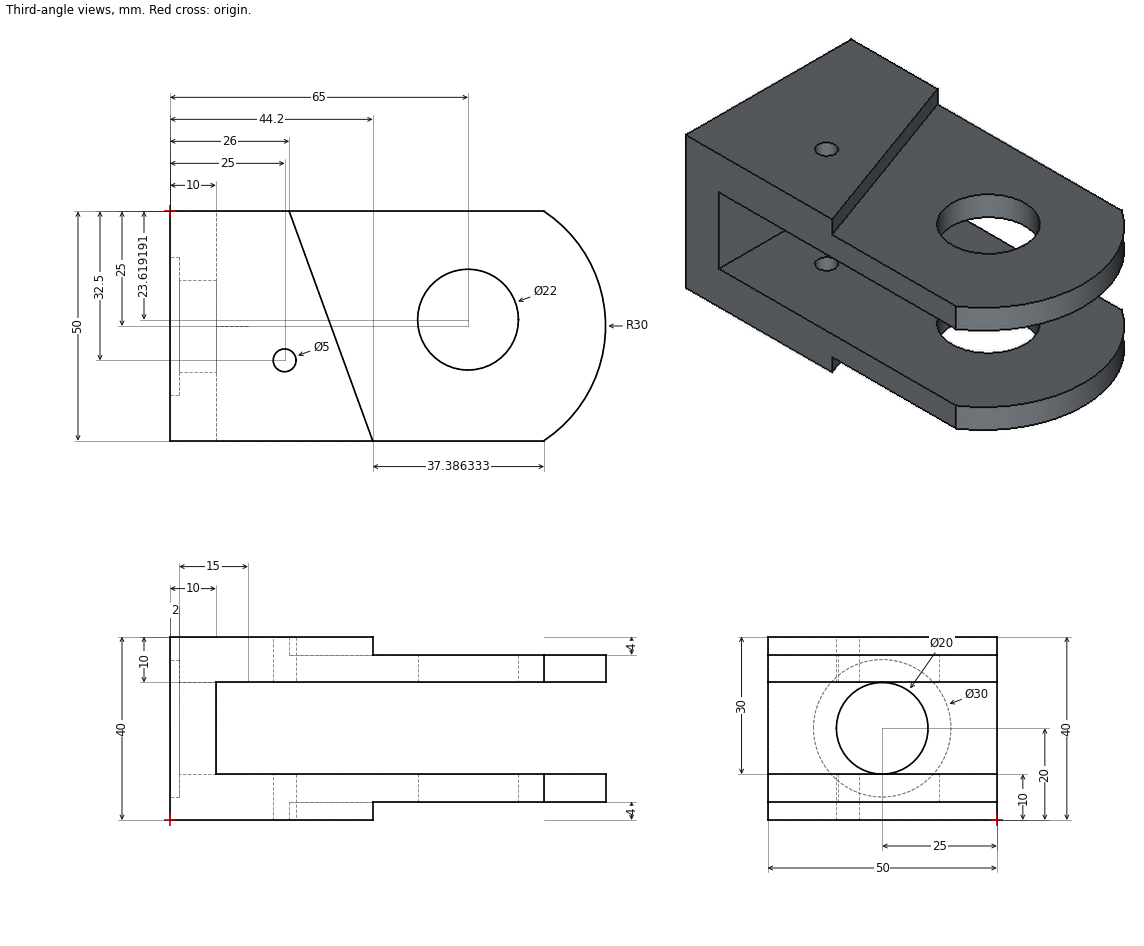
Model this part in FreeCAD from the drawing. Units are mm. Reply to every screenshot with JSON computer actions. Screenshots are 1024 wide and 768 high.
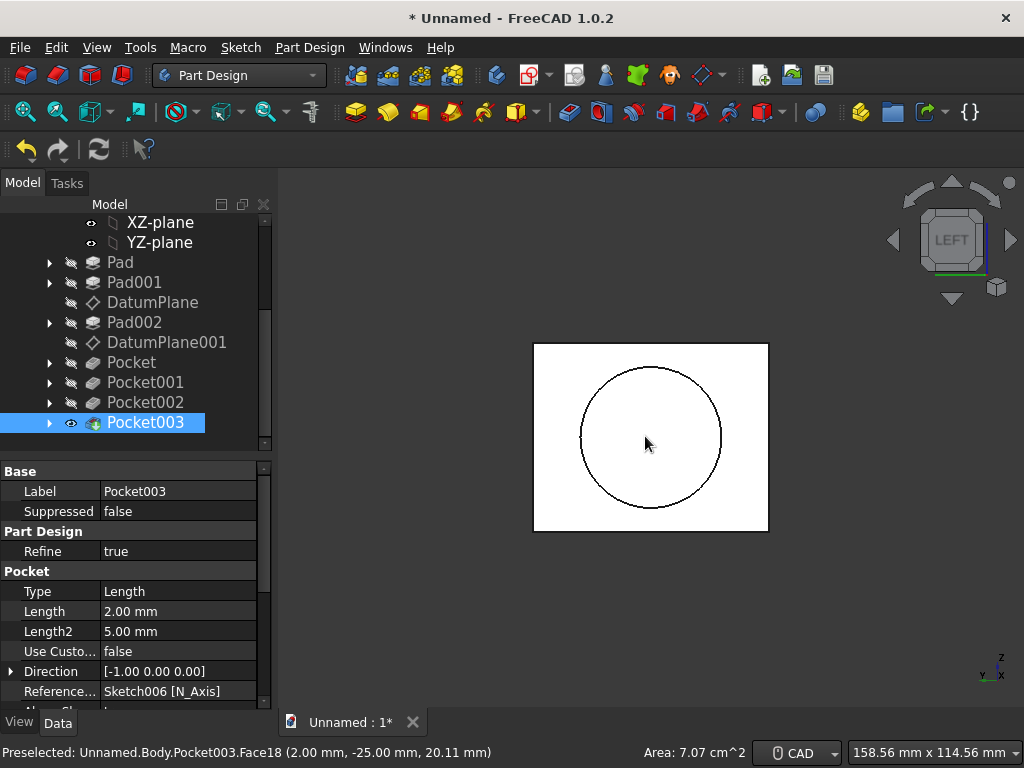
{"action": "left_click", "coordinate": [530, 76]}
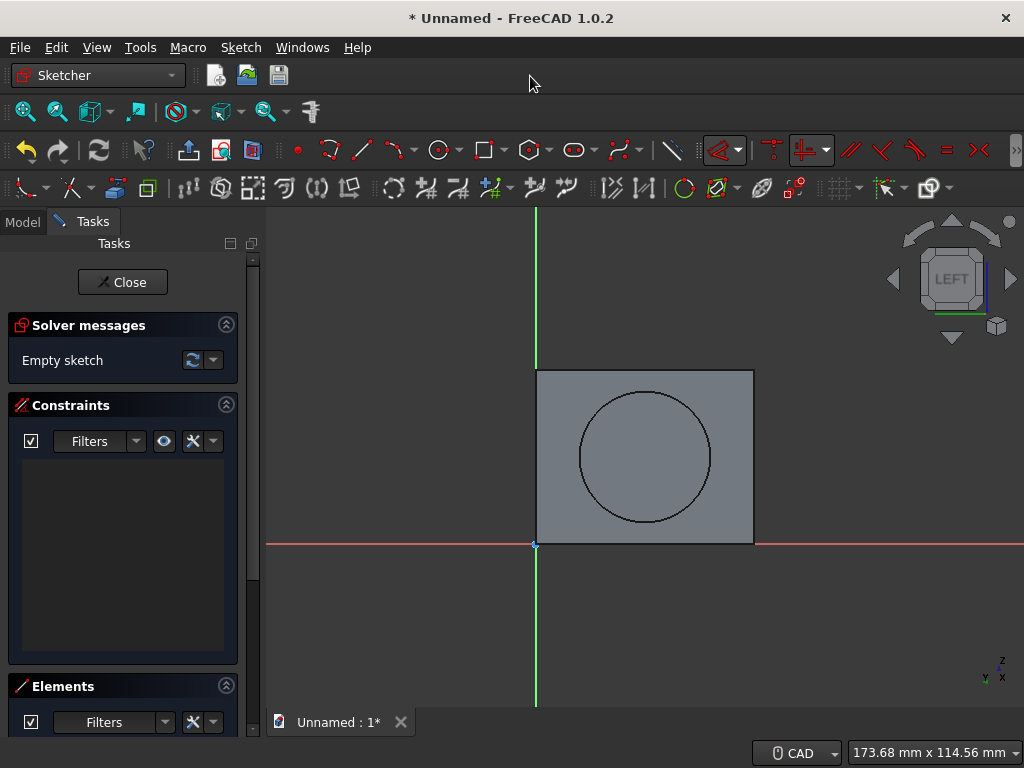
{"action": "left_click", "coordinate": [254, 150]}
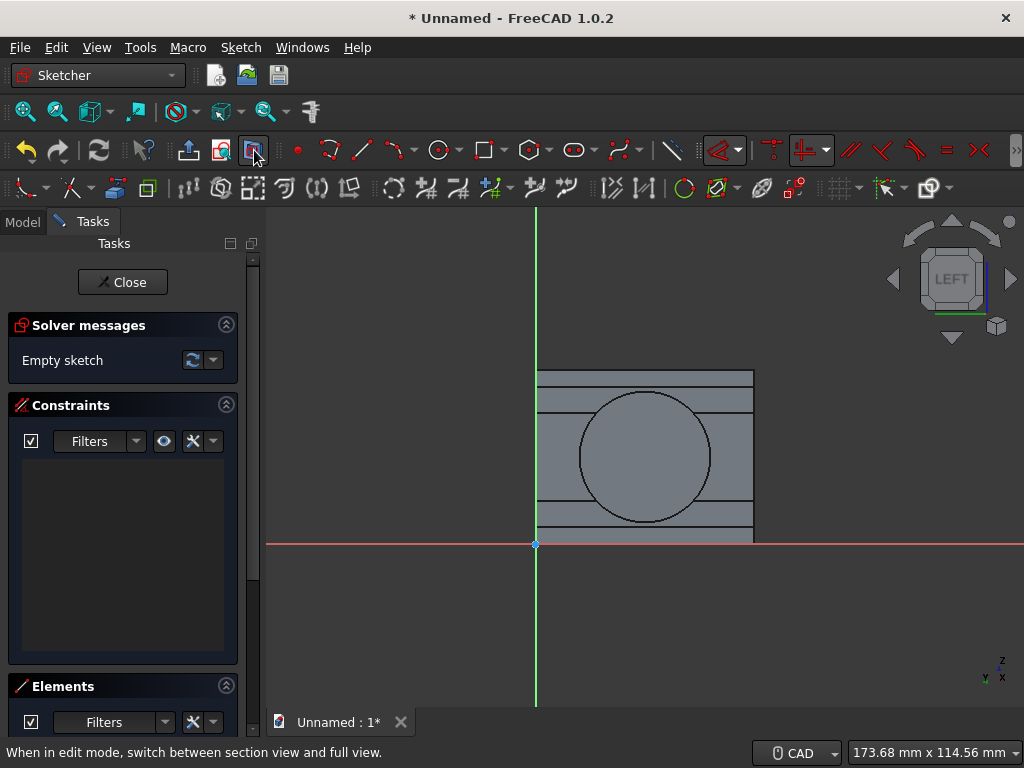
{"action": "scroll", "coordinate": [641, 497], "scroll_direction": "up", "scroll_amount": 4}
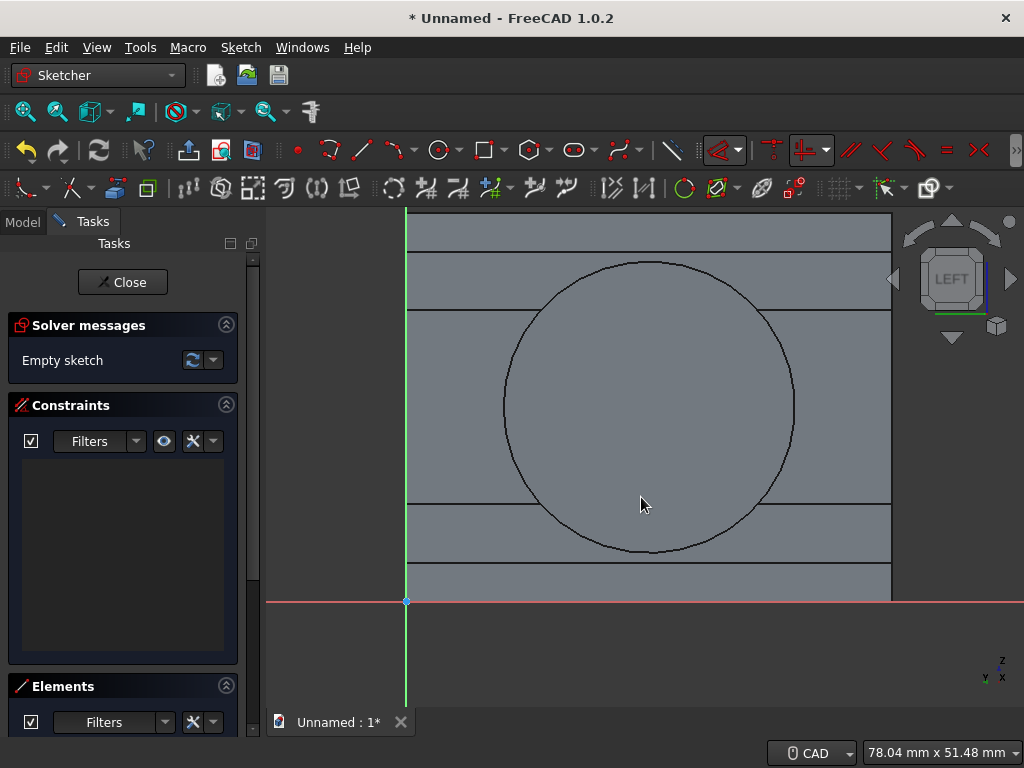
{"action": "left_click", "coordinate": [440, 150]}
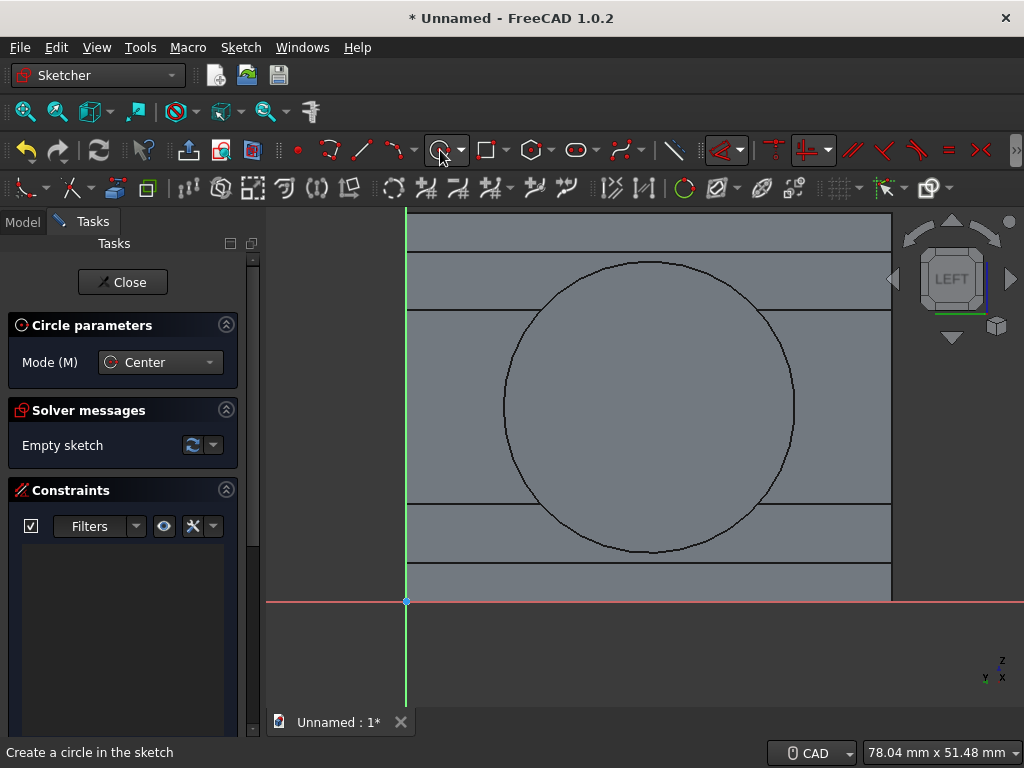
{"action": "left_click", "coordinate": [649, 407]}
{"action": "mouse_move", "coordinate": [718, 339]}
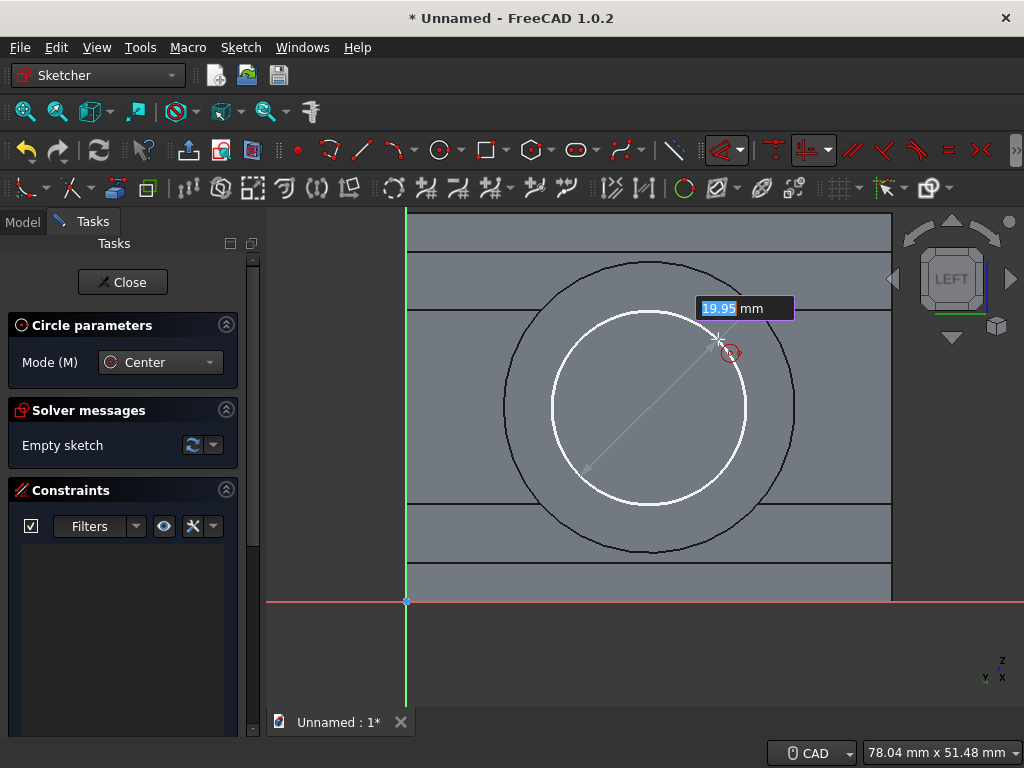
{"action": "type", "text": "20"}
{"action": "key", "text": "Return"}
{"action": "key", "text": "Escape"}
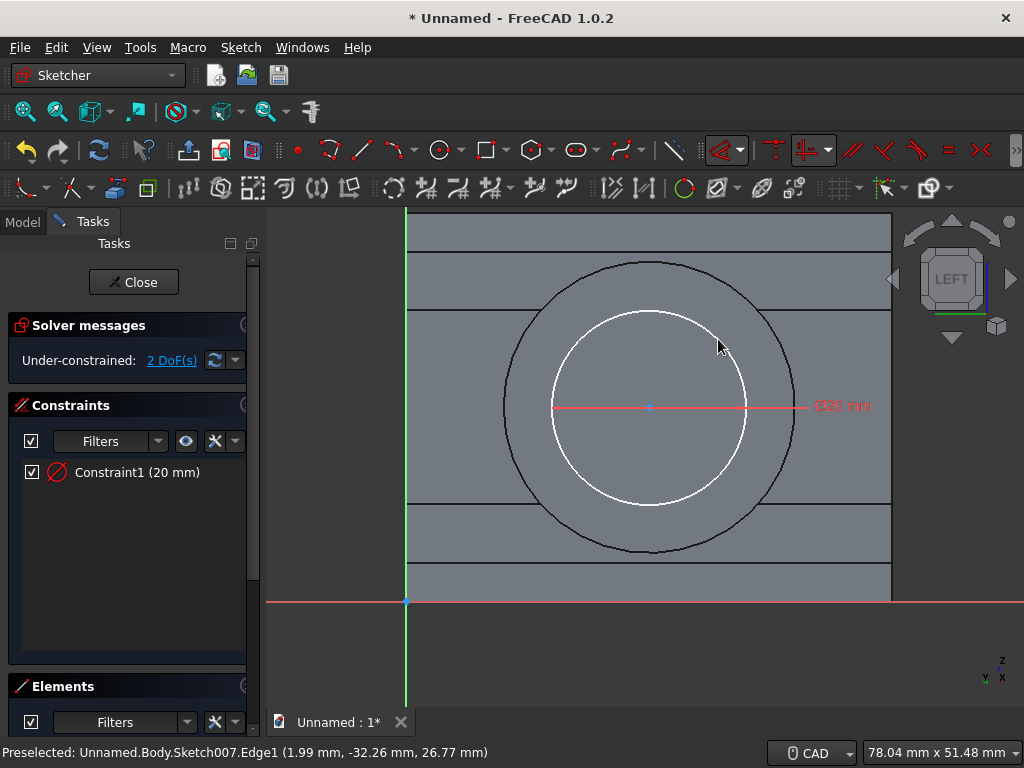
{"action": "left_click", "coordinate": [649, 408]}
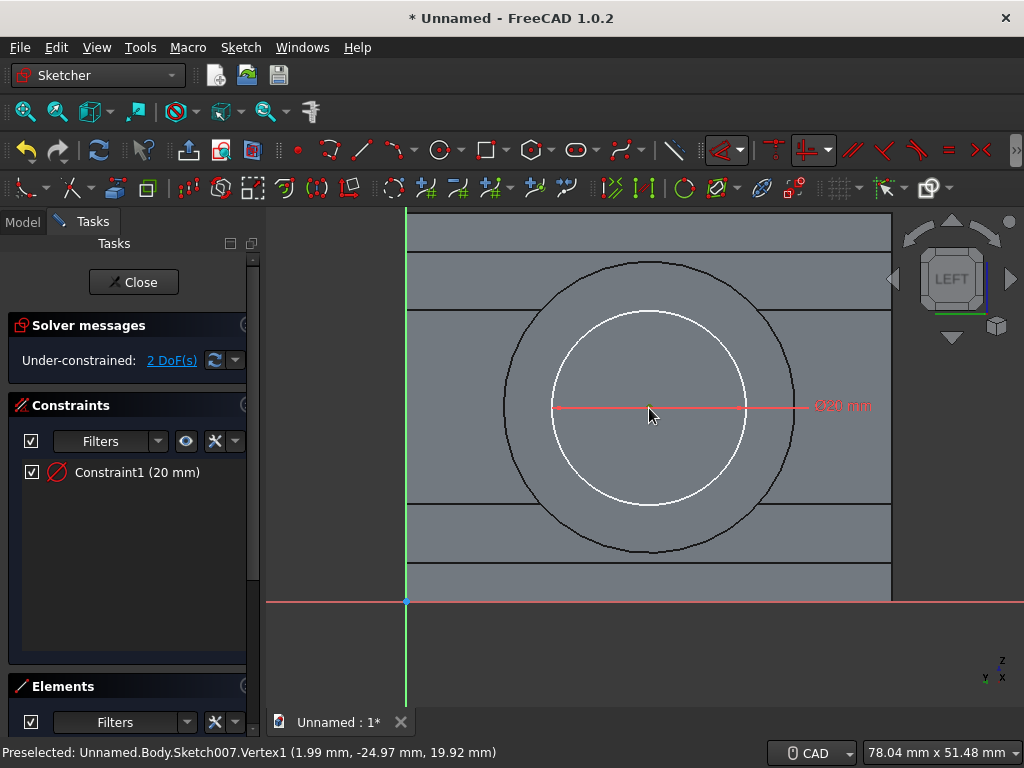
{"action": "left_click", "coordinate": [742, 150]}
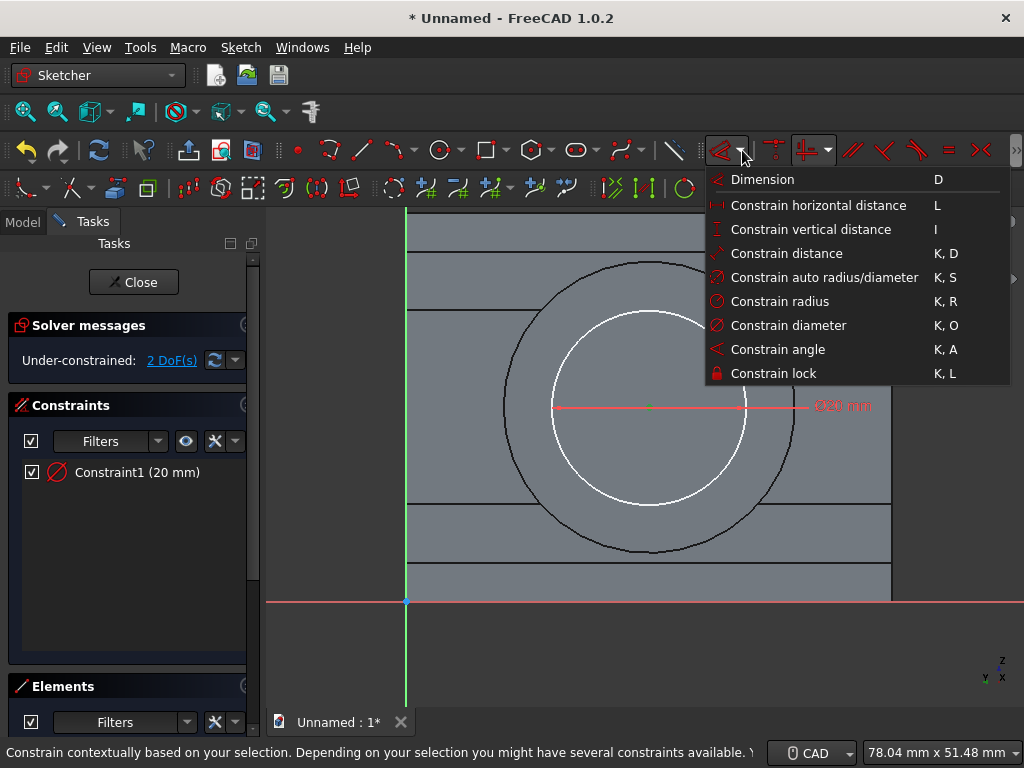
{"action": "left_click", "coordinate": [858, 205]}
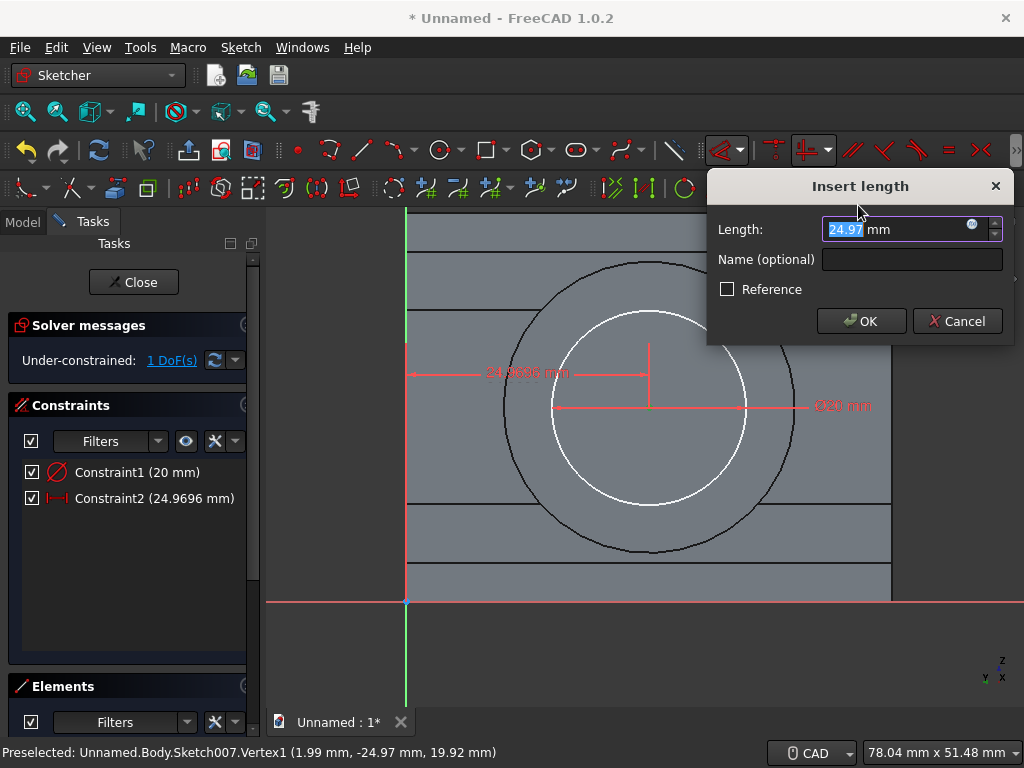
{"action": "type", "text": "25"}
{"action": "key", "text": "Return"}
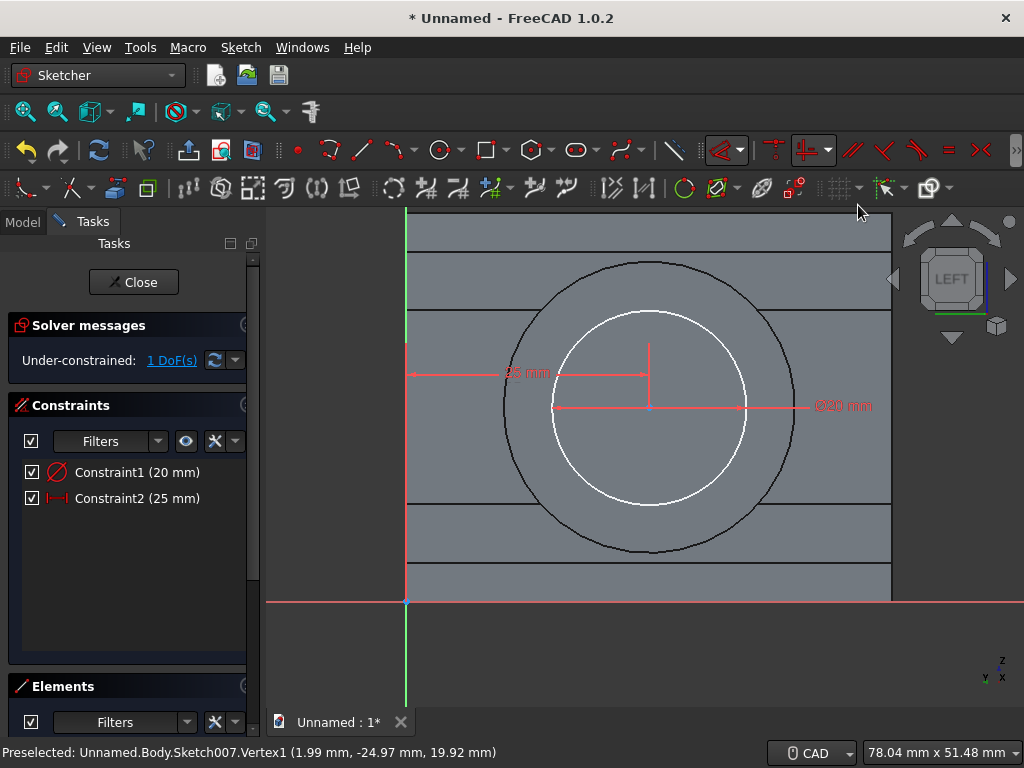
{"action": "left_click", "coordinate": [649, 408]}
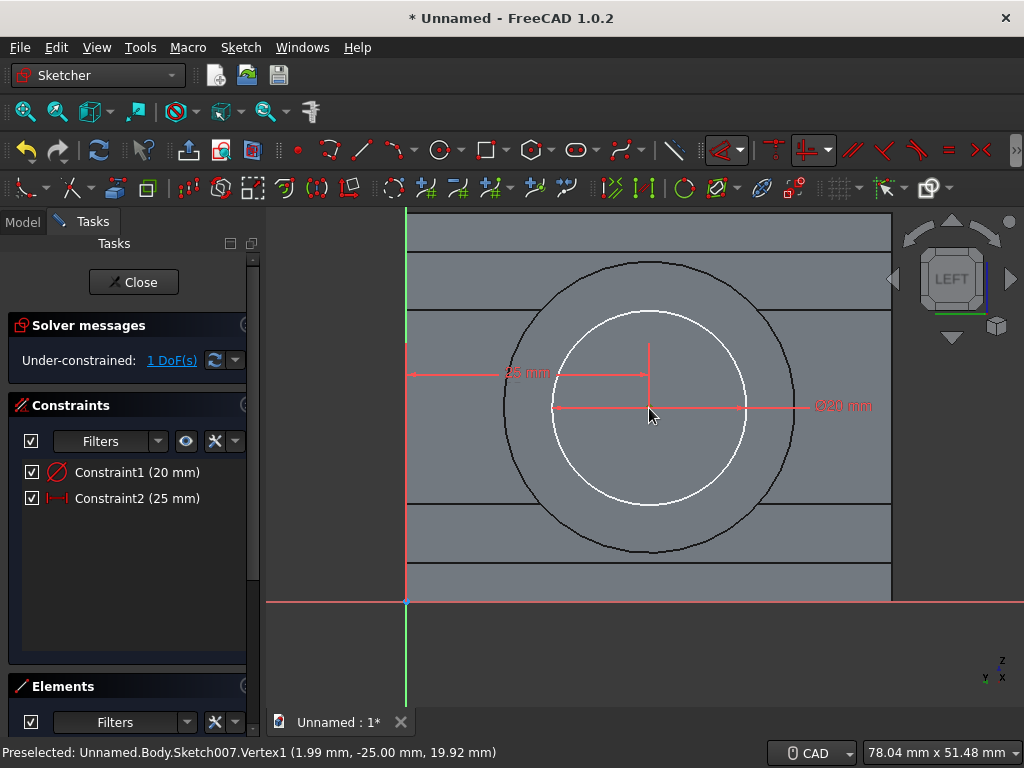
{"action": "key", "text": "i"}